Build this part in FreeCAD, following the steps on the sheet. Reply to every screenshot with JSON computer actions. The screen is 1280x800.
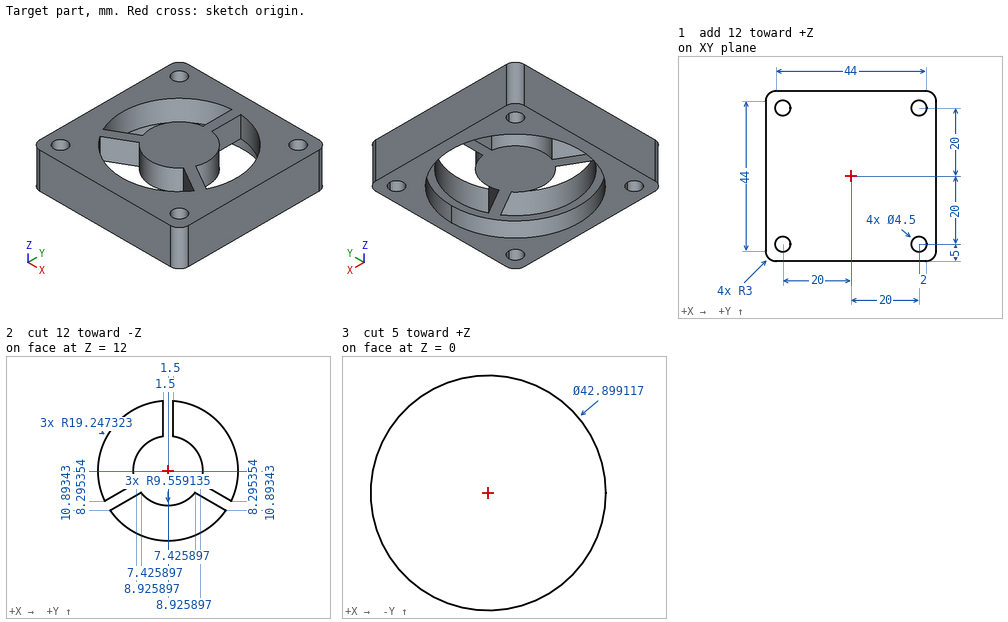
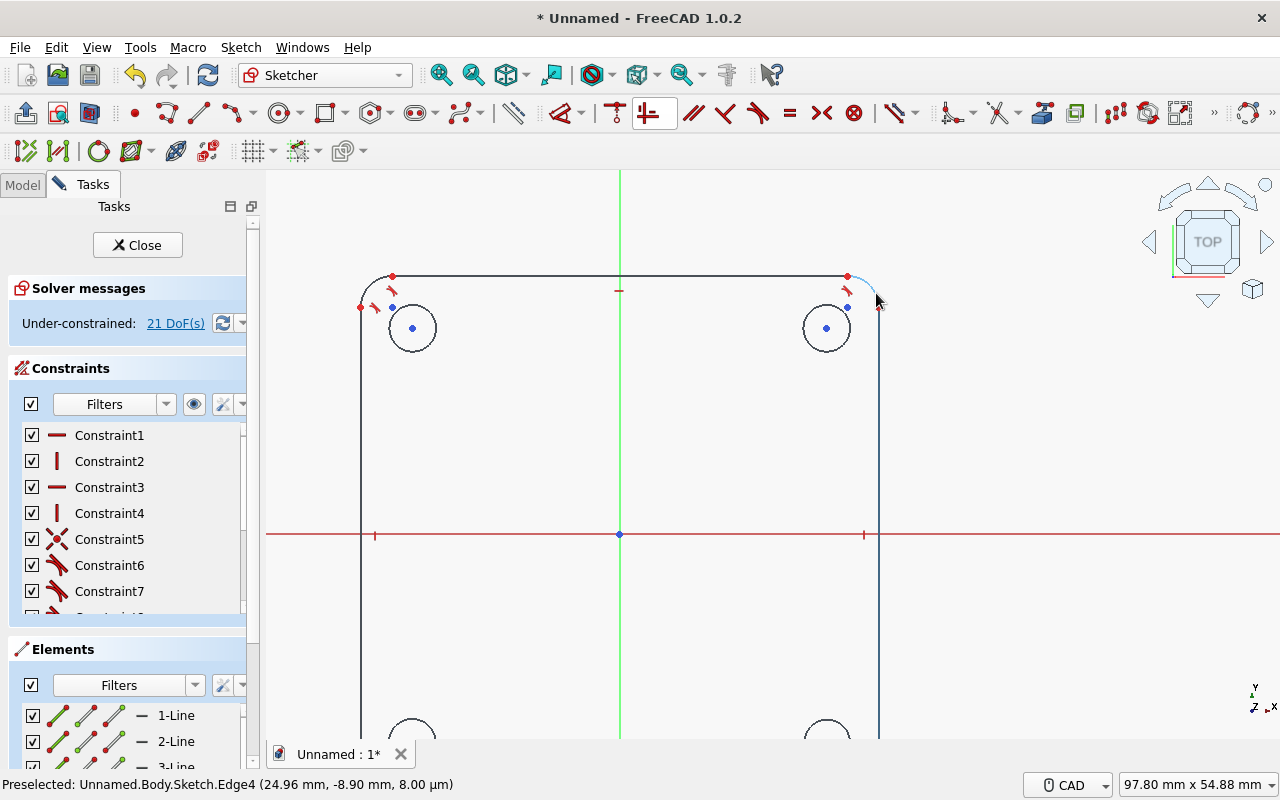
{"action": "left_click", "coordinate": [875, 293]}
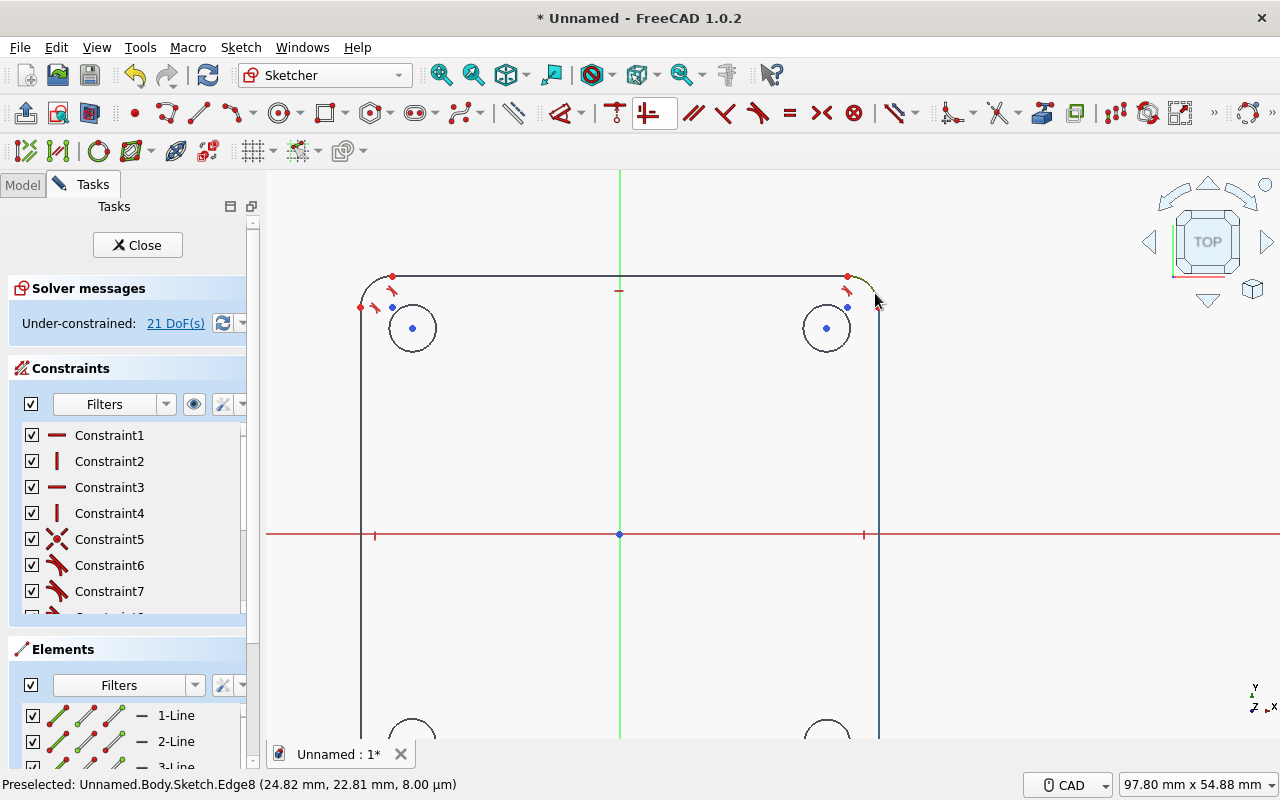
{"action": "left_click", "coordinate": [758, 114]}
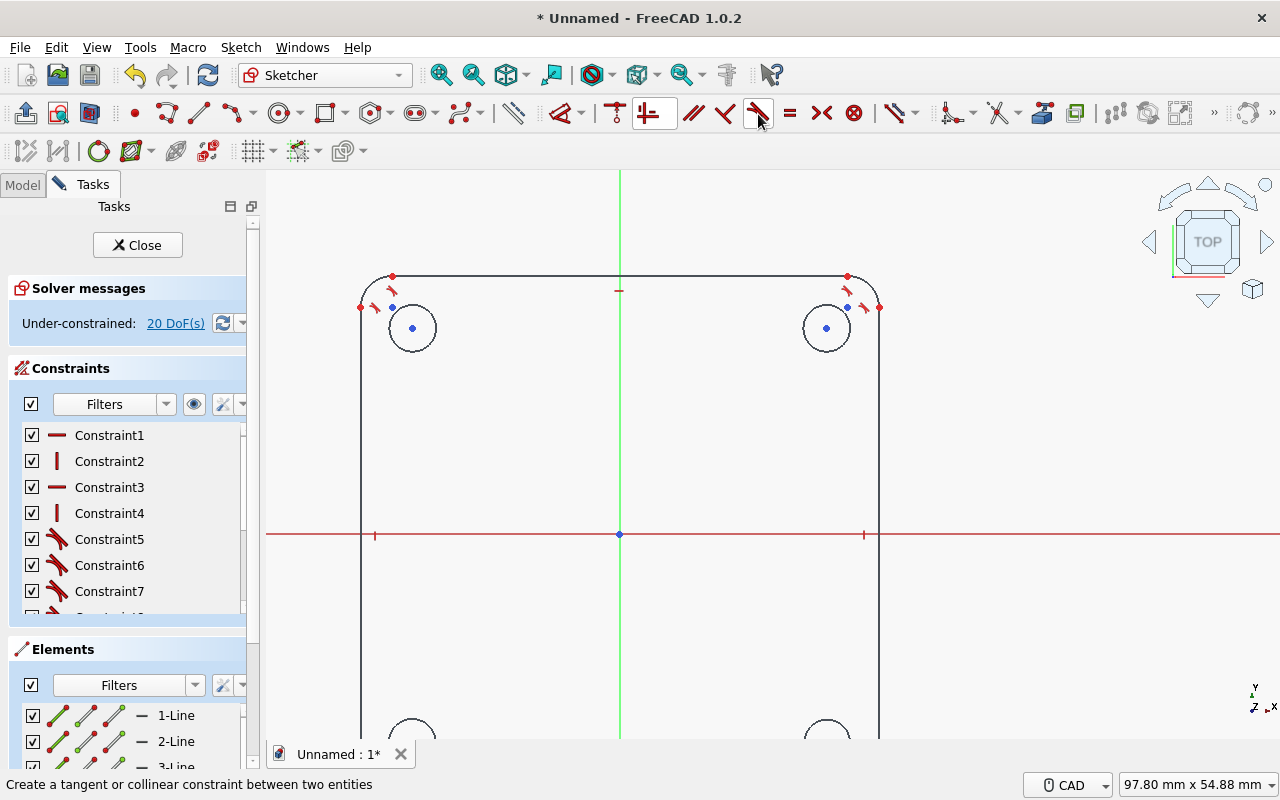
{"action": "left_click", "coordinate": [378, 280]}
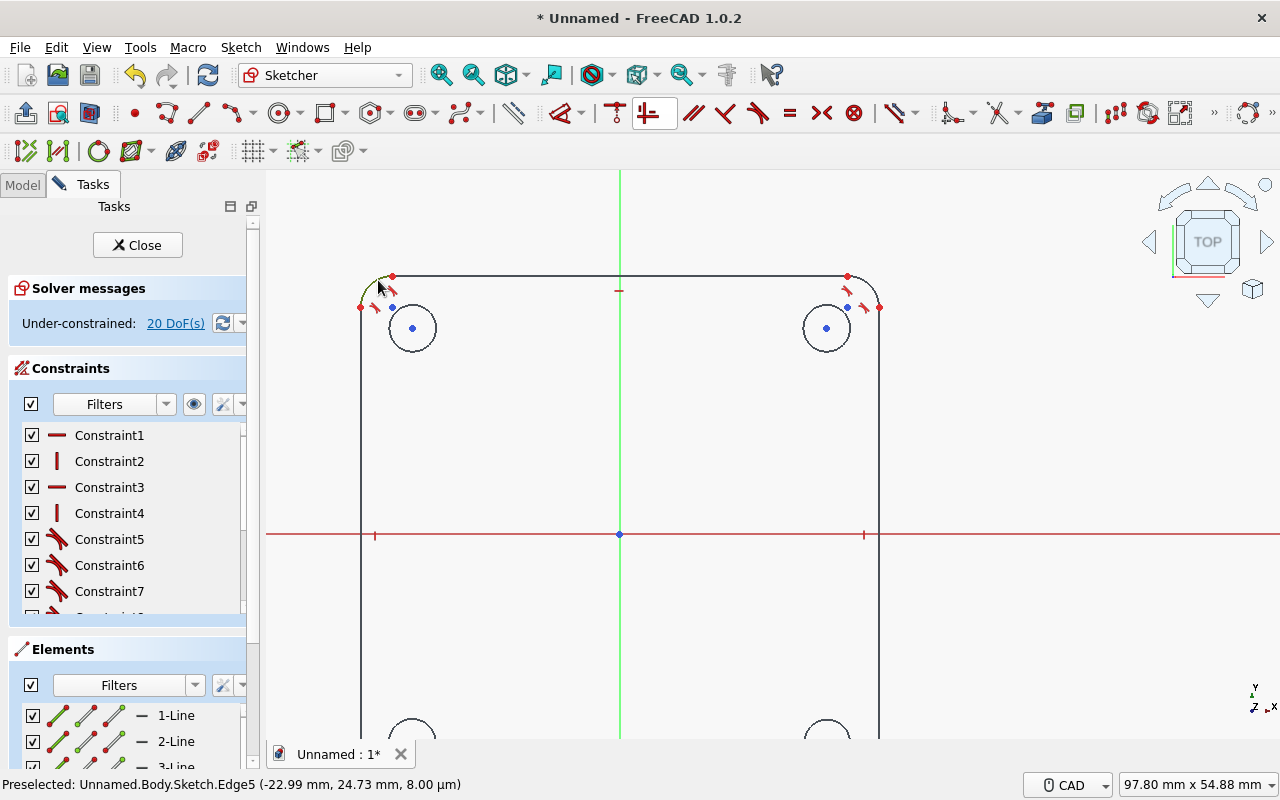
{"action": "scroll", "coordinate": [877, 292], "scroll_direction": "down", "scroll_amount": 2}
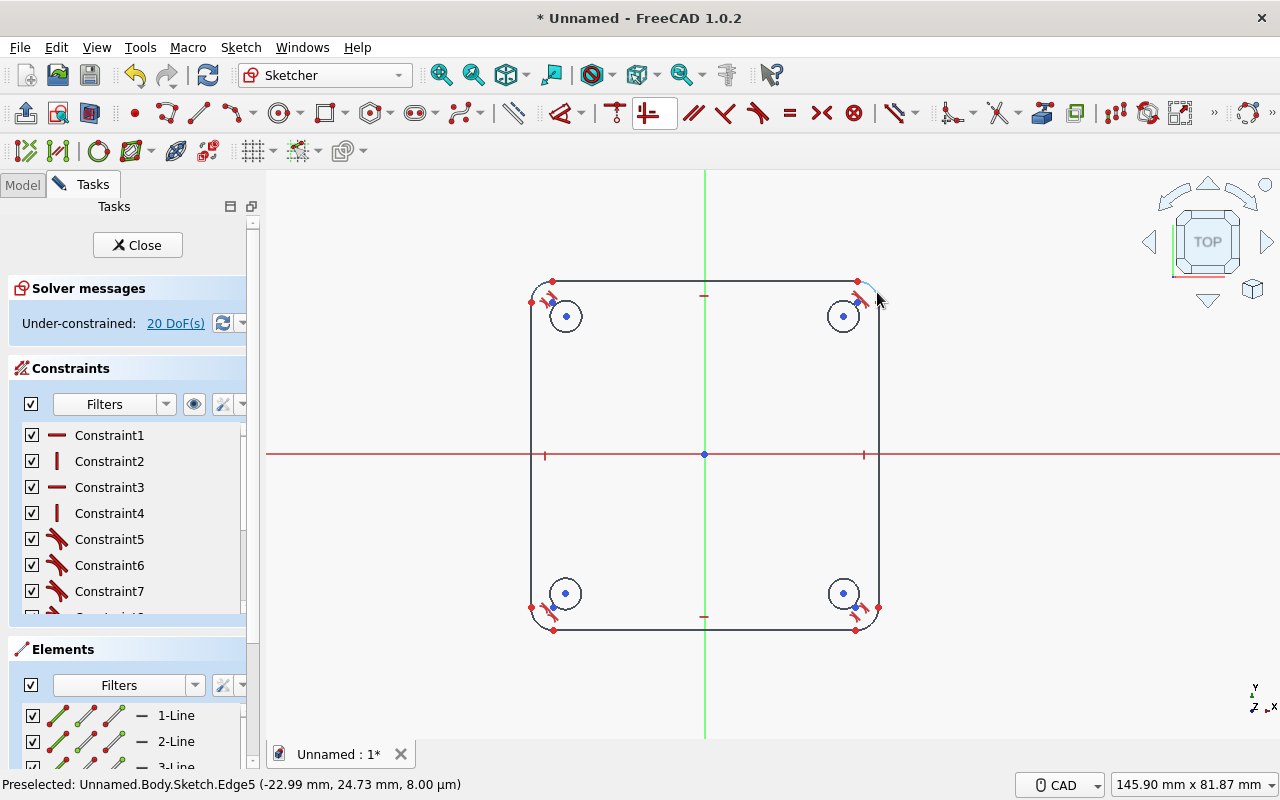
{"action": "scroll", "coordinate": [534, 618], "scroll_direction": "up", "scroll_amount": 2}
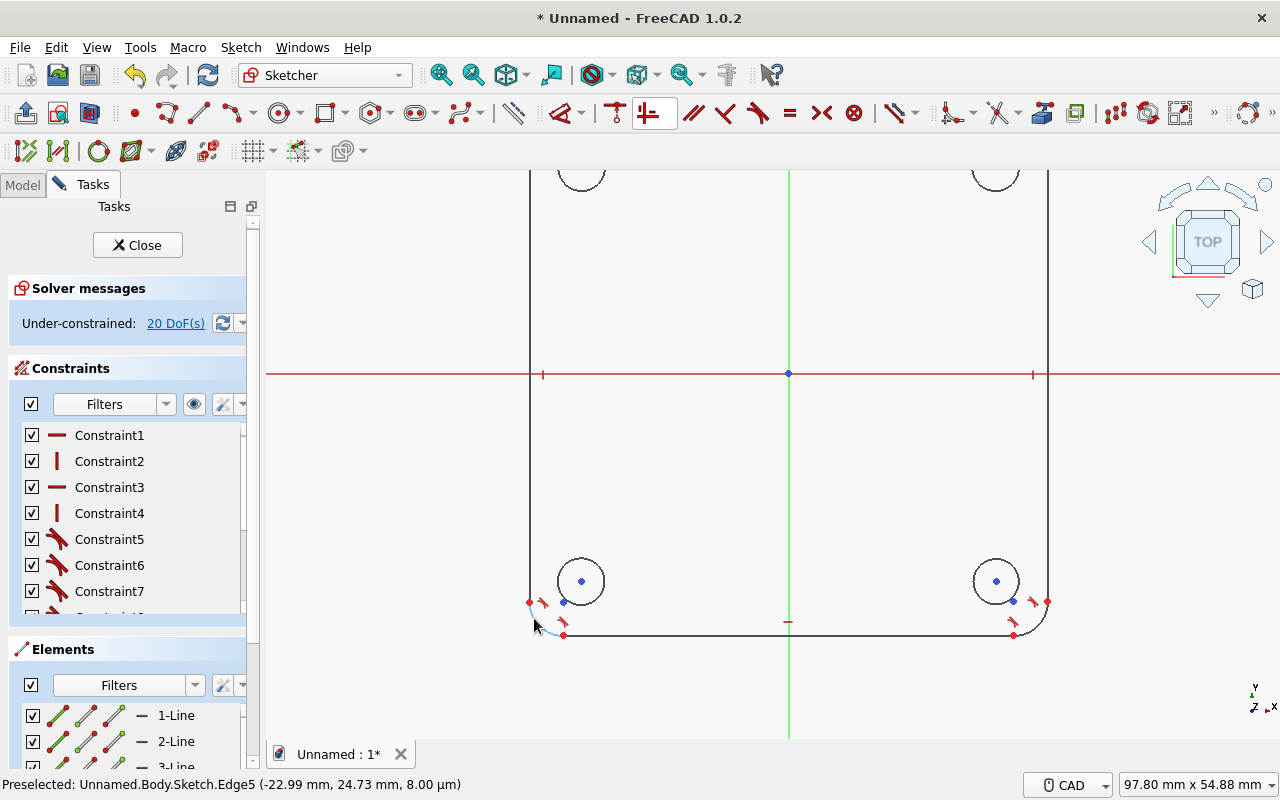
{"action": "left_click", "coordinate": [533, 618]}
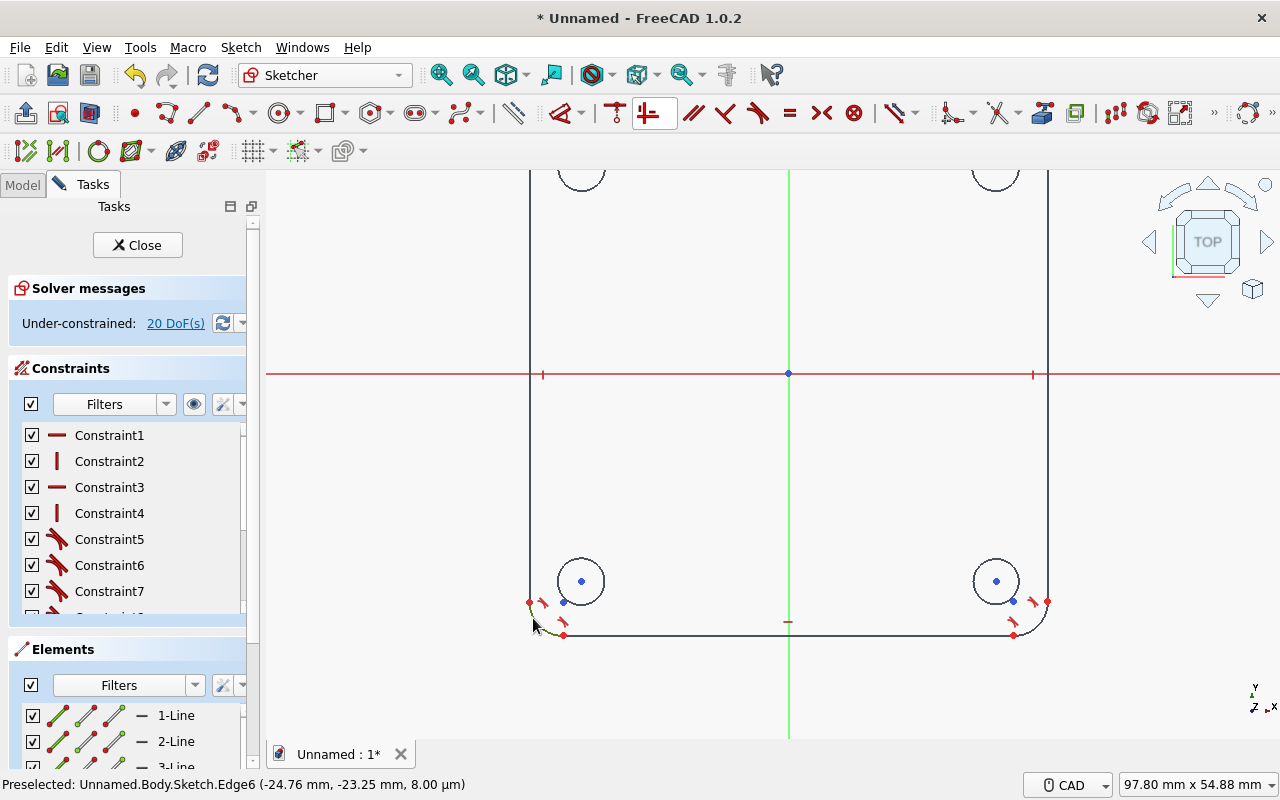
{"action": "left_click", "coordinate": [1029, 632]}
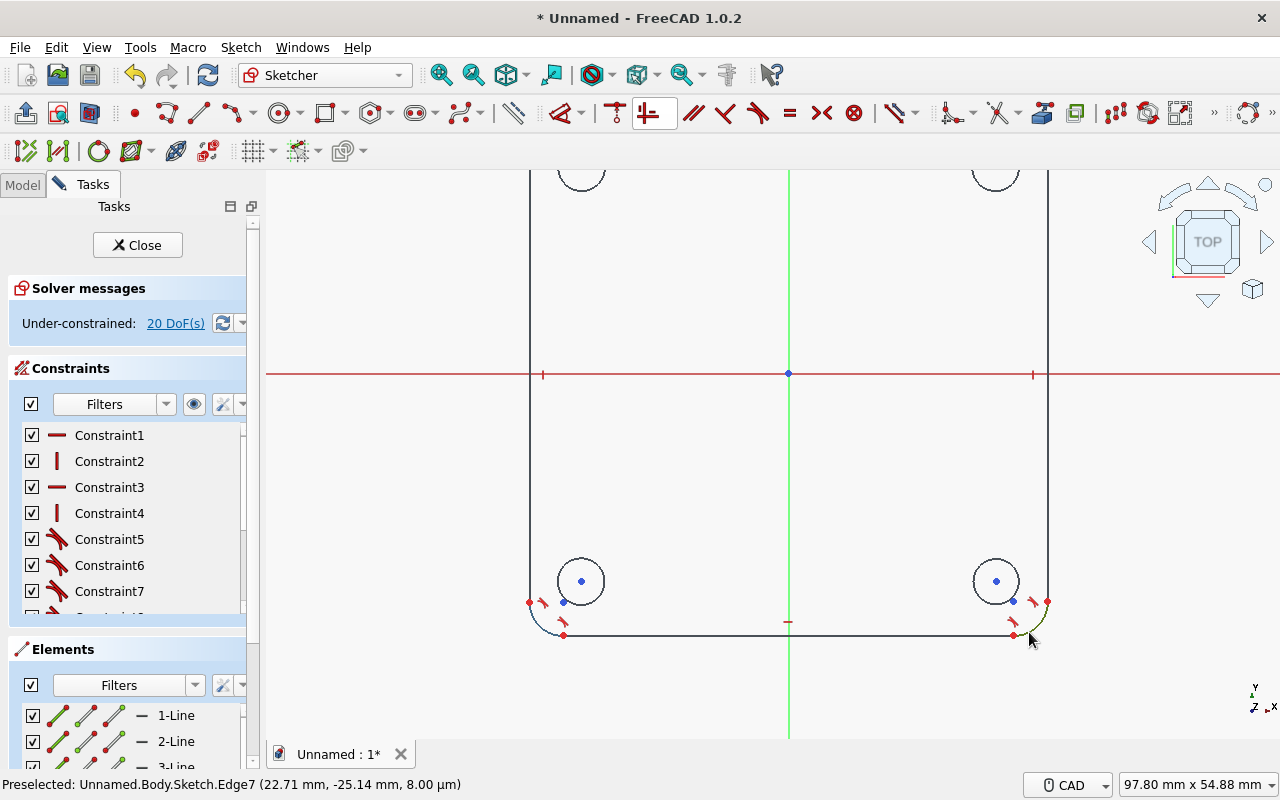
{"action": "scroll", "coordinate": [533, 619], "scroll_direction": "down", "scroll_amount": 2}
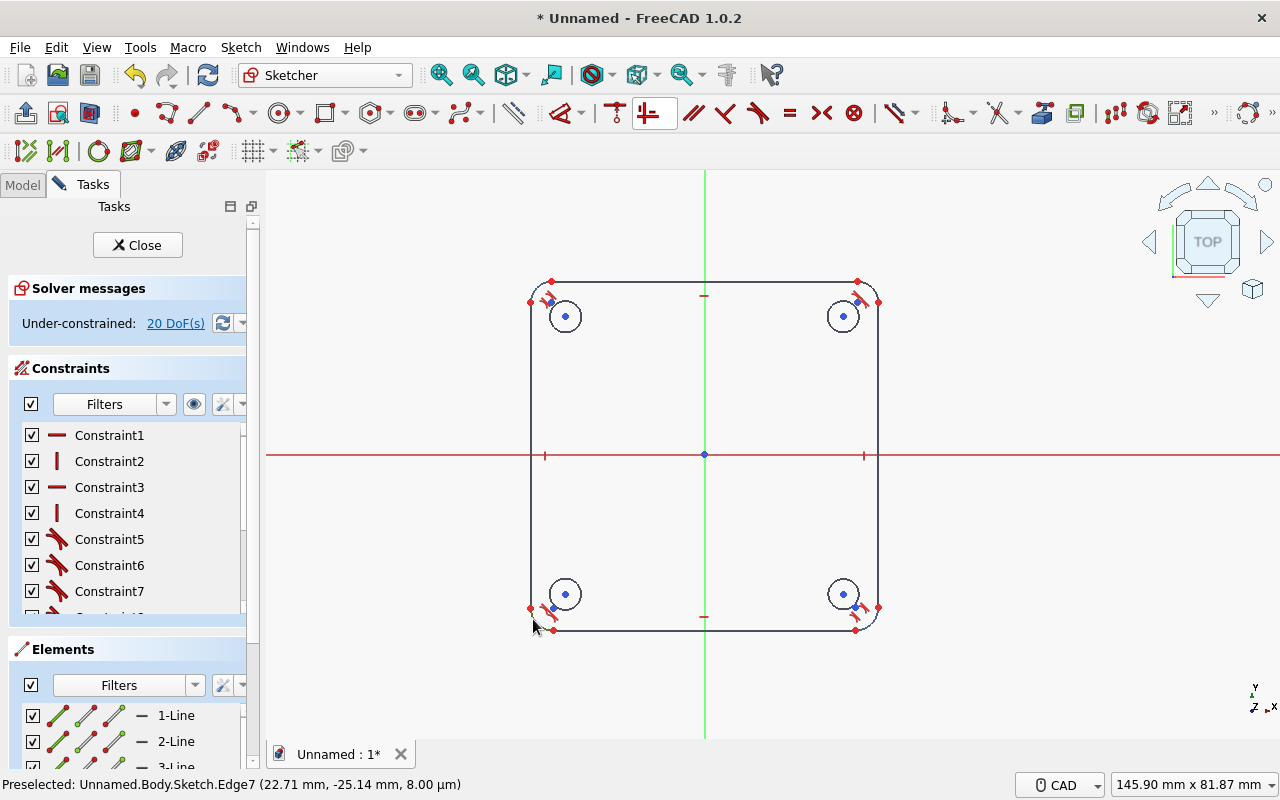
{"action": "scroll", "coordinate": [876, 293], "scroll_direction": "up", "scroll_amount": 2}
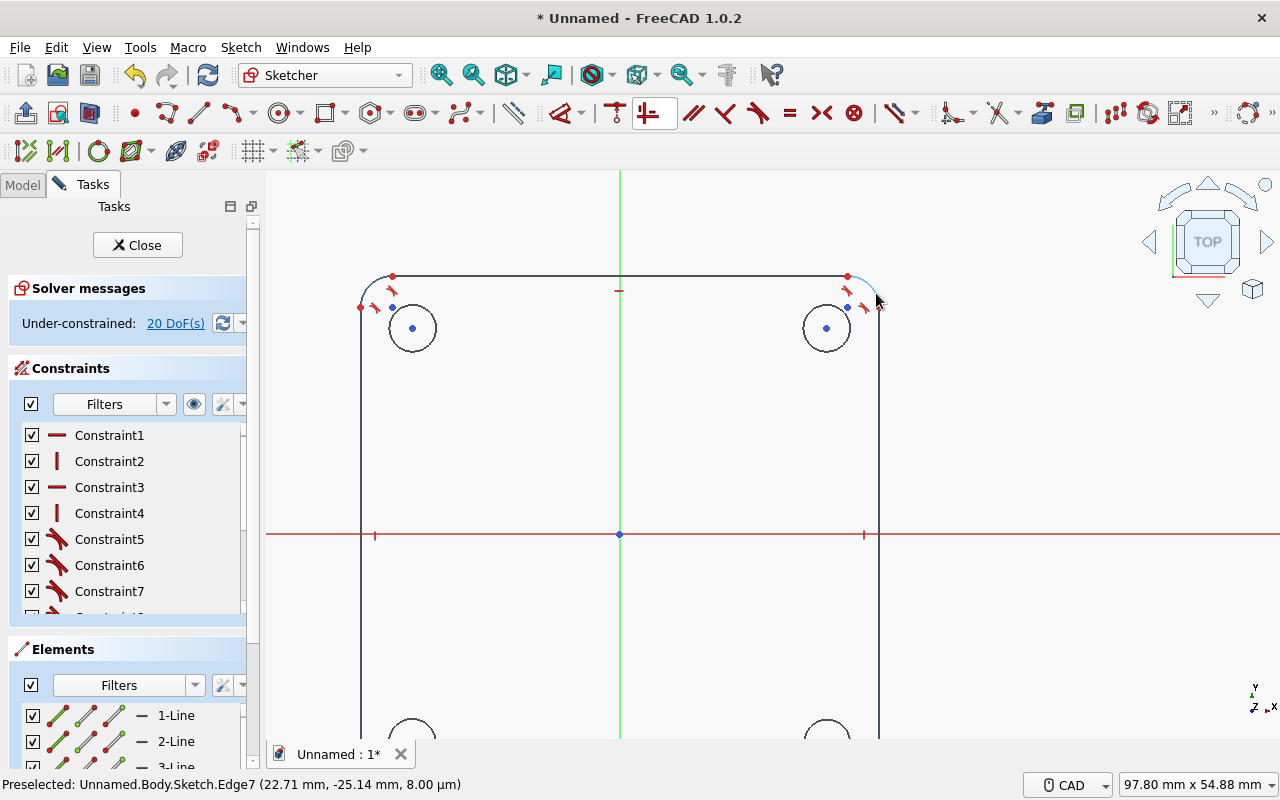
{"action": "left_click", "coordinate": [876, 293]}